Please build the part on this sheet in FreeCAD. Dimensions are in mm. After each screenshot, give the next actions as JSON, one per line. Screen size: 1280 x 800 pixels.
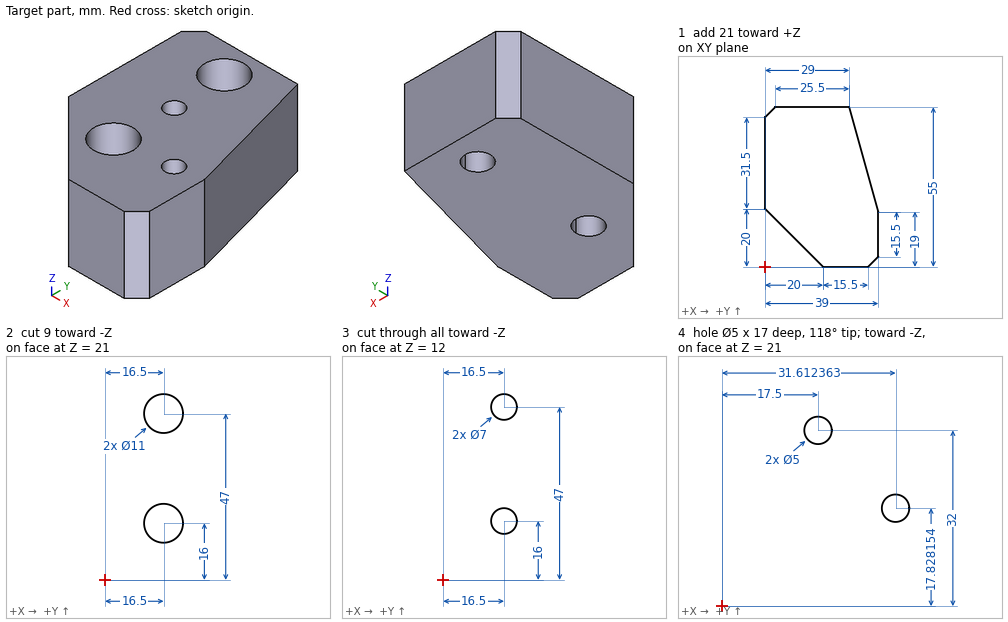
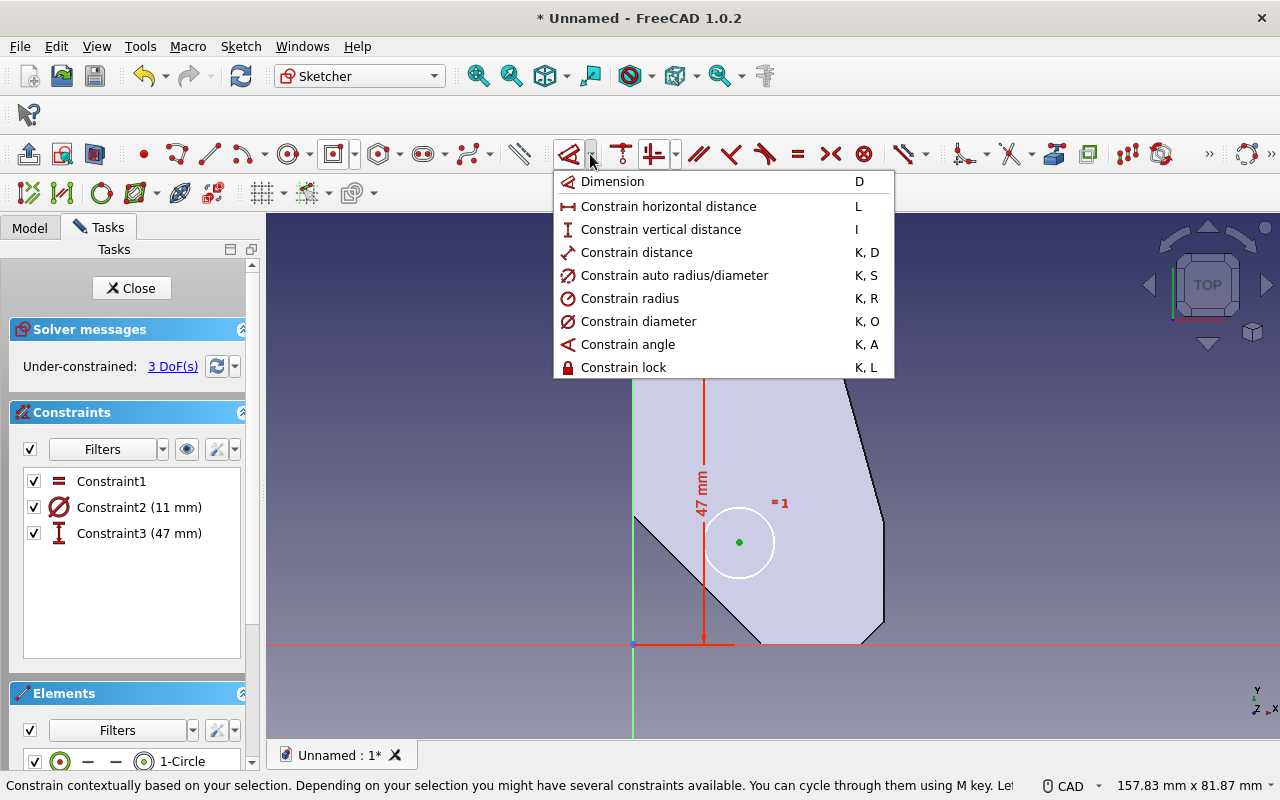
{"action": "left_click", "coordinate": [724, 230]}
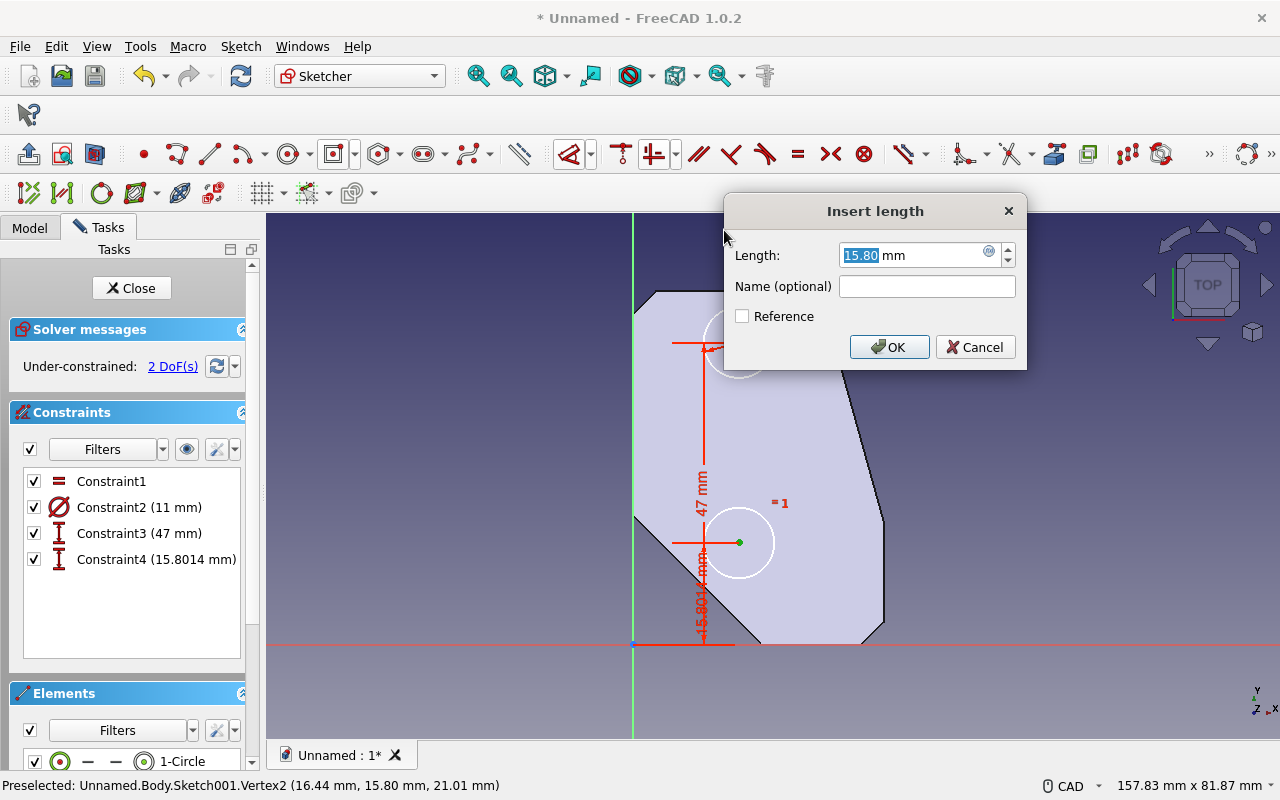
{"action": "type", "text": "16"}
{"action": "key", "text": "Return"}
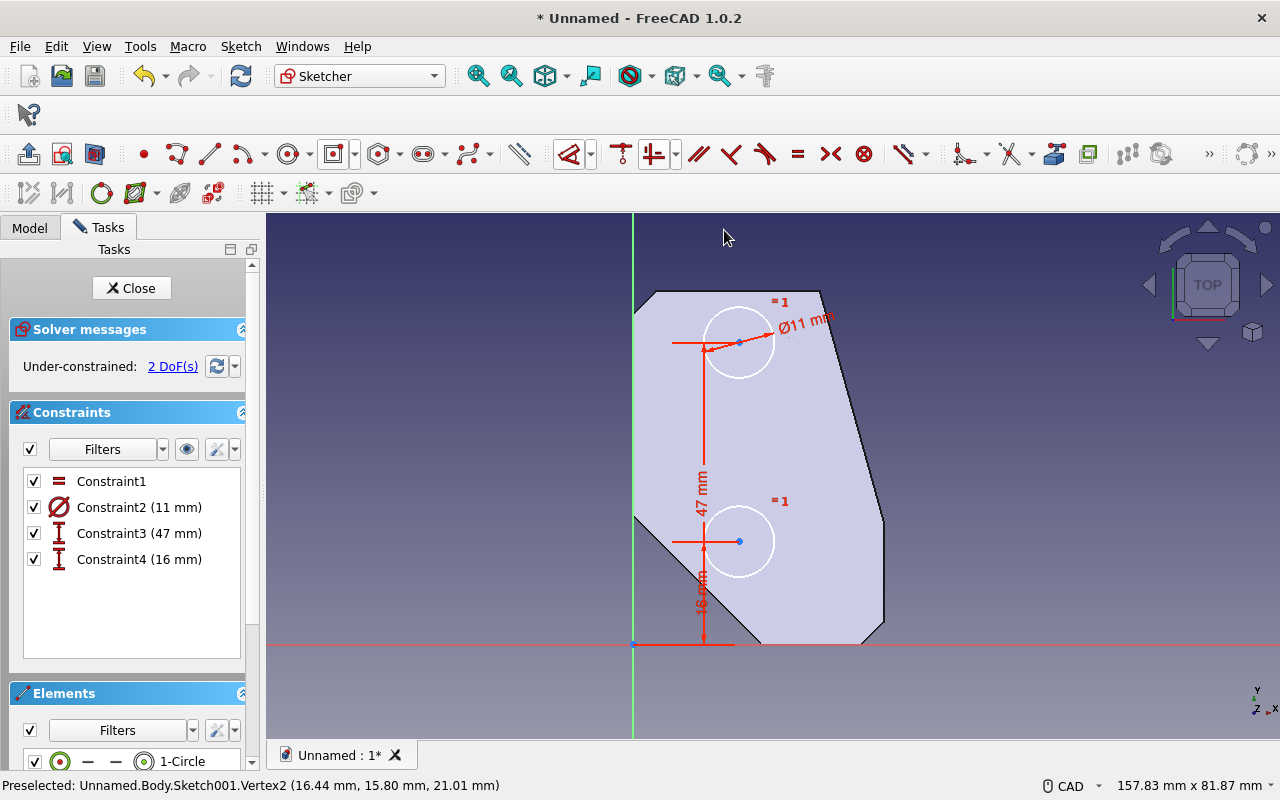
{"action": "left_click", "coordinate": [739, 343]}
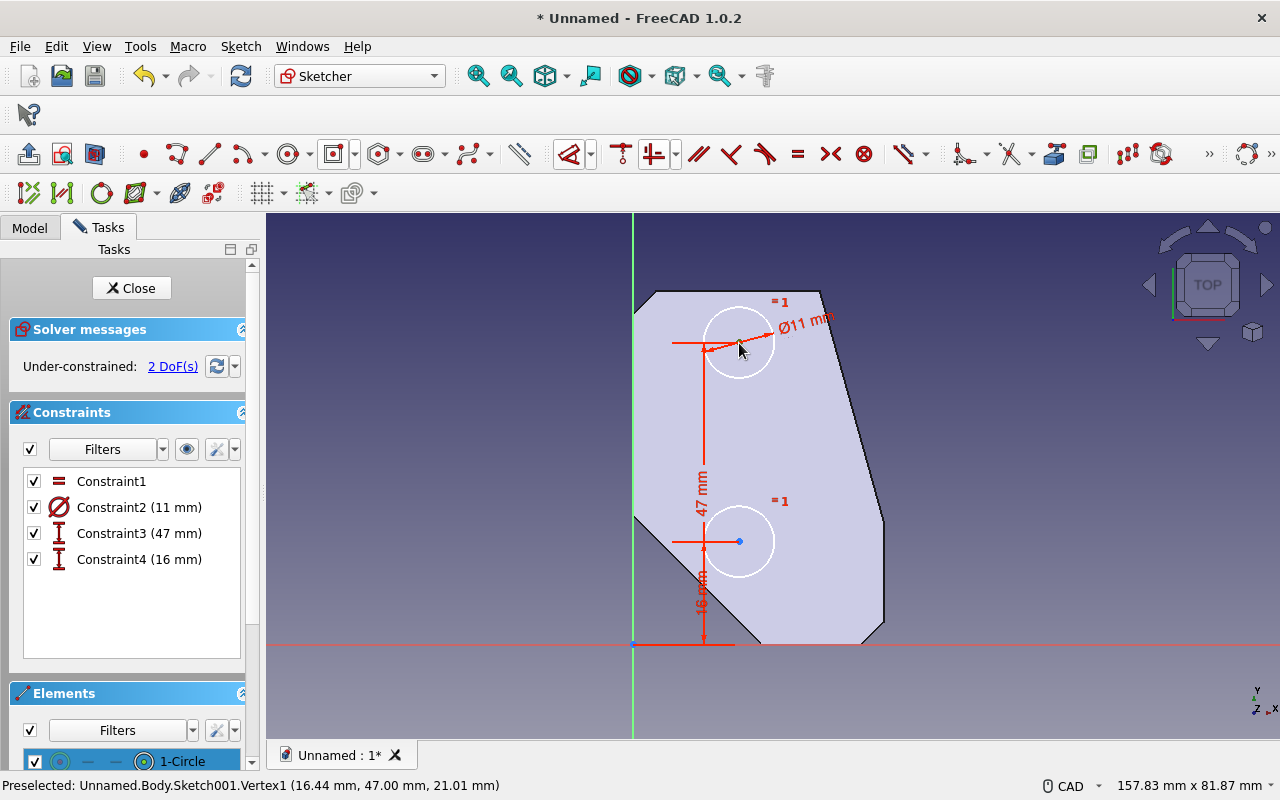
{"action": "key", "text": "l"}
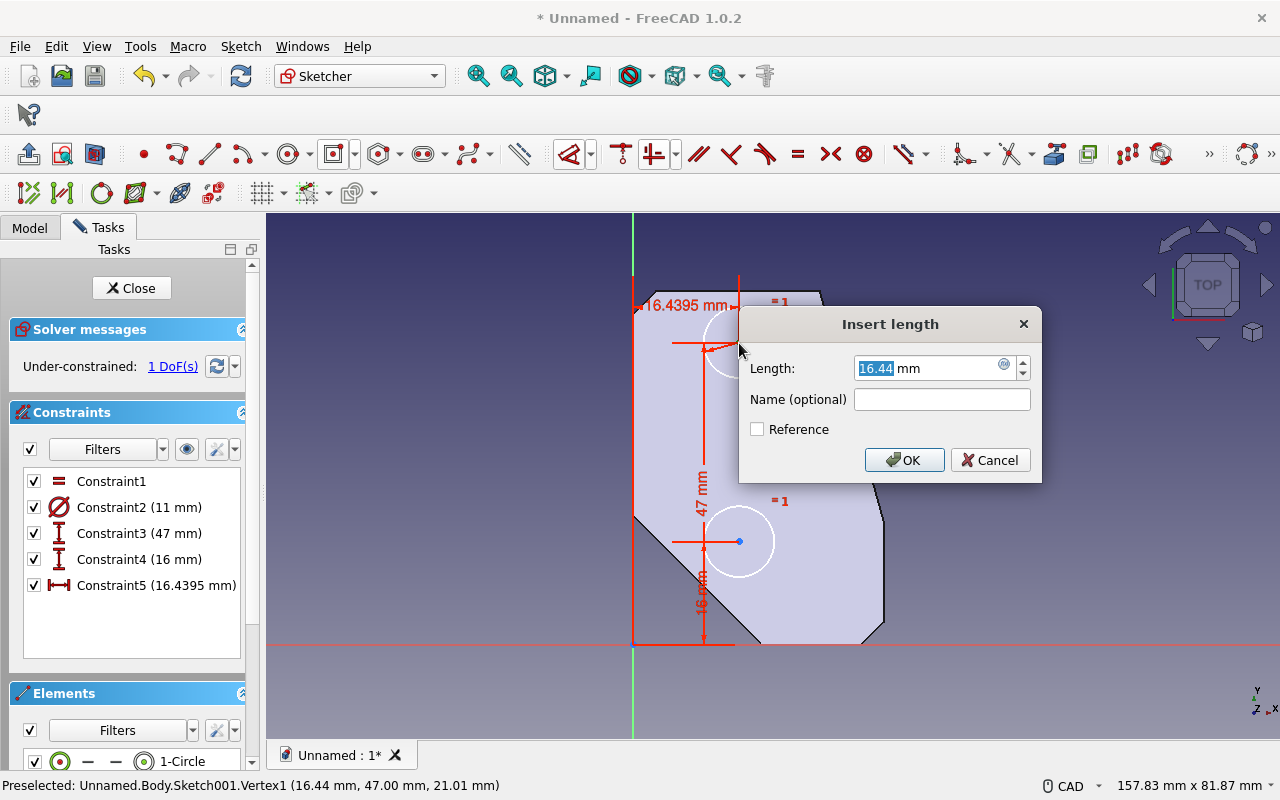
{"action": "type", "text": "16.5"}
{"action": "key", "text": "Return"}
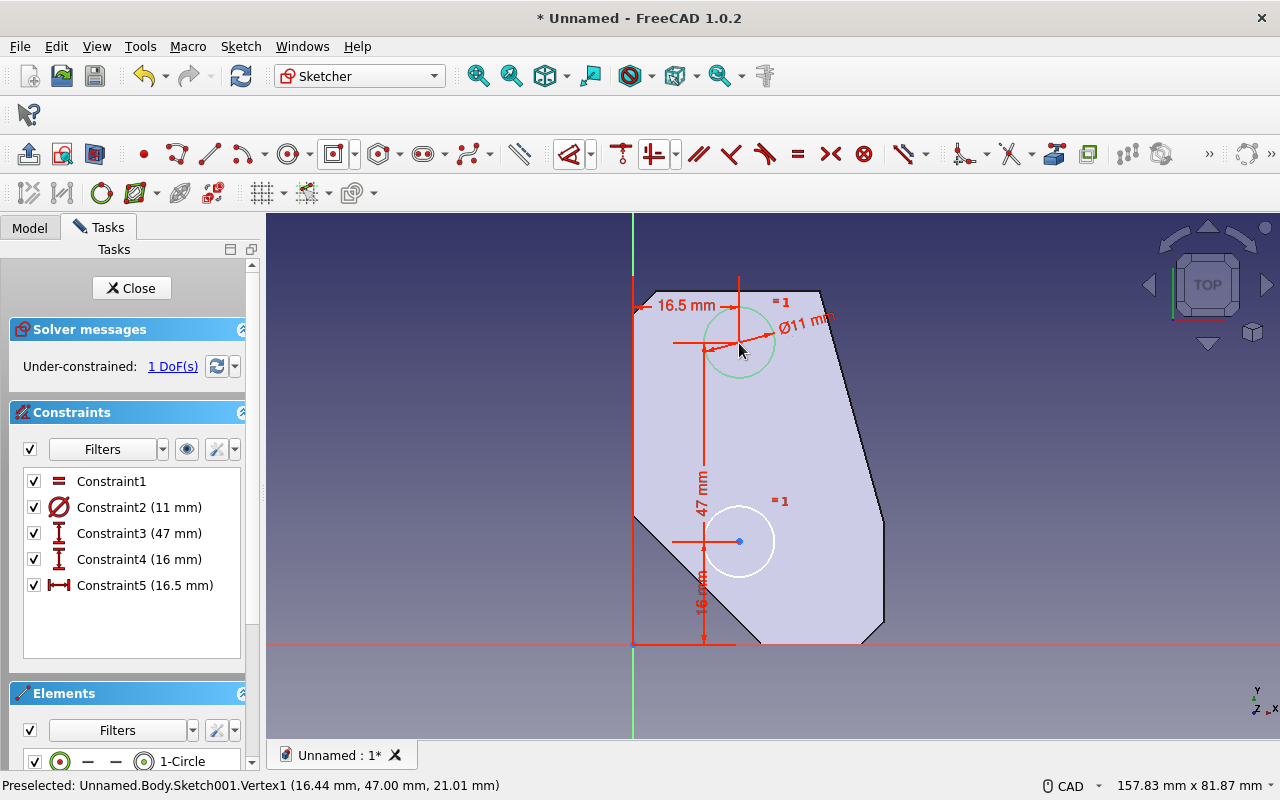
{"action": "left_click", "coordinate": [739, 542]}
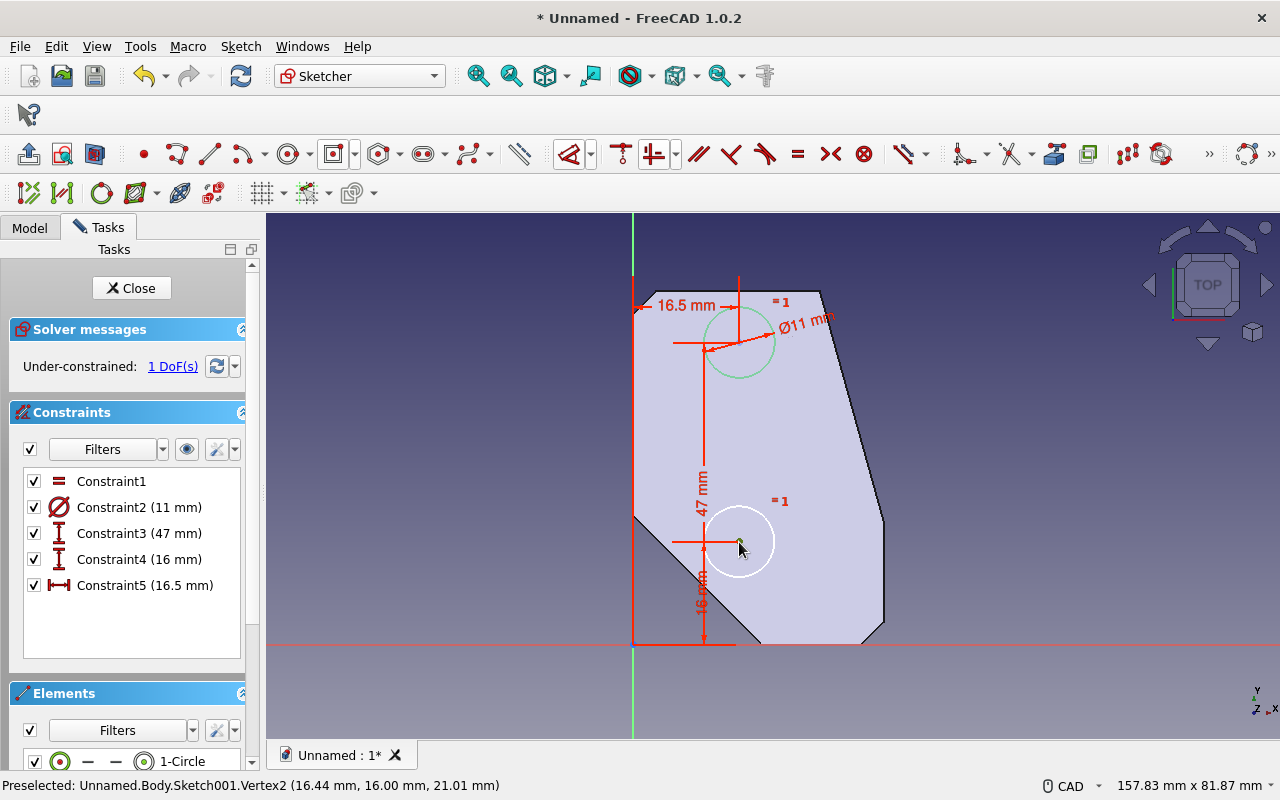
{"action": "key", "text": "l"}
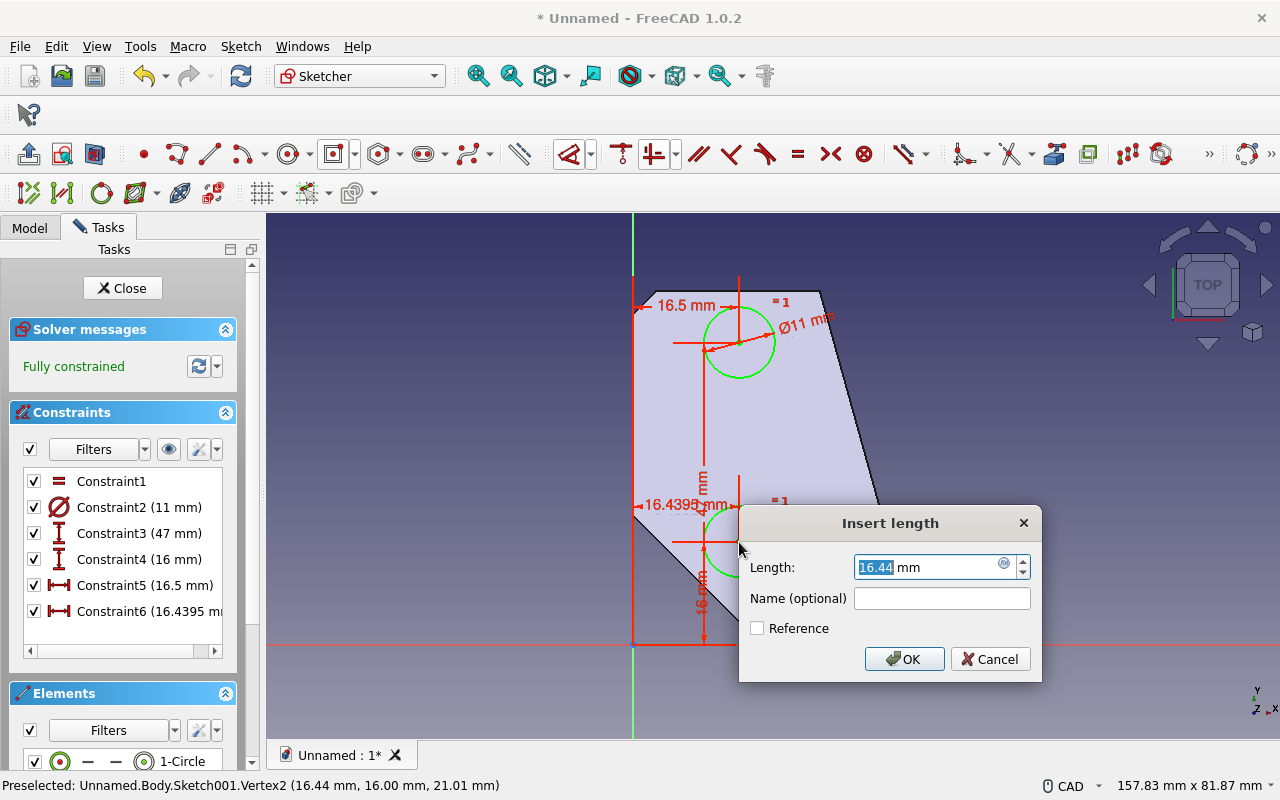
{"action": "type", "text": "16.5"}
{"action": "key", "text": "Return"}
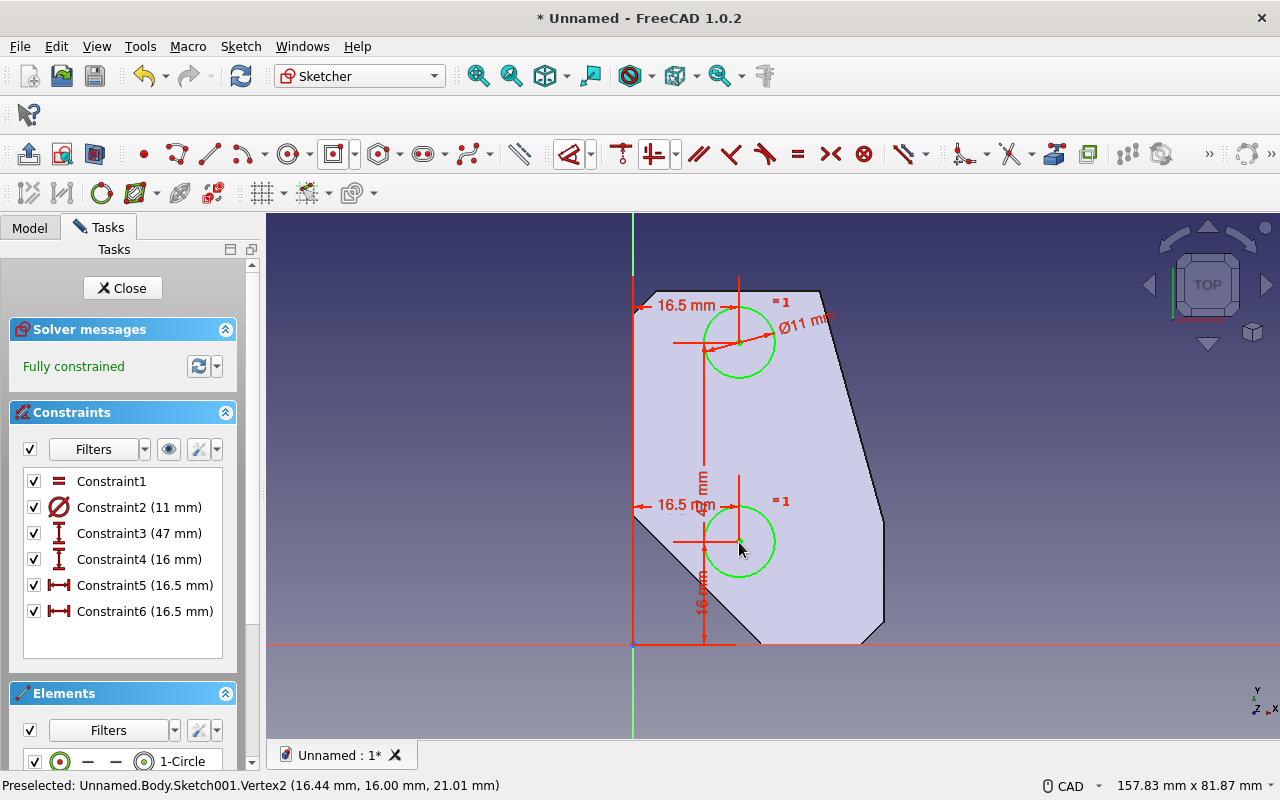
{"action": "left_click", "coordinate": [123, 288]}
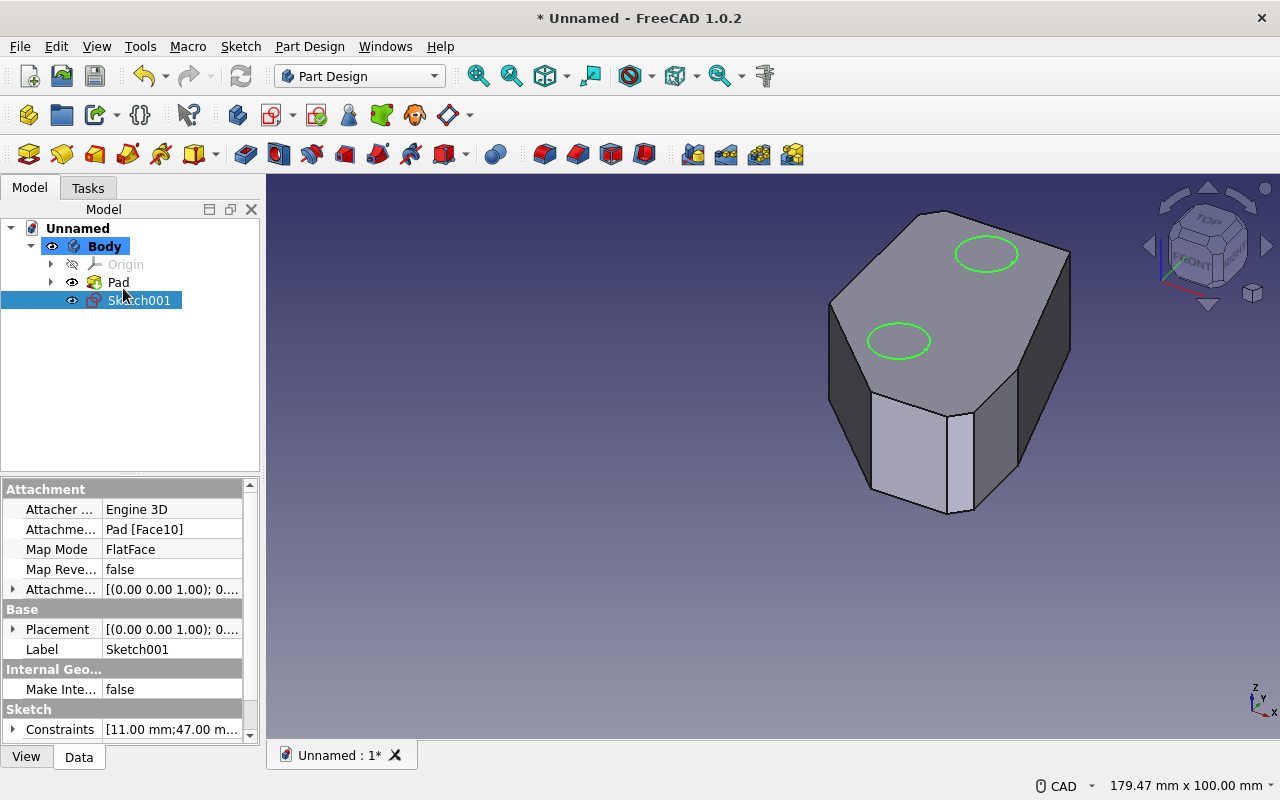
{"action": "left_click", "coordinate": [246, 154]}